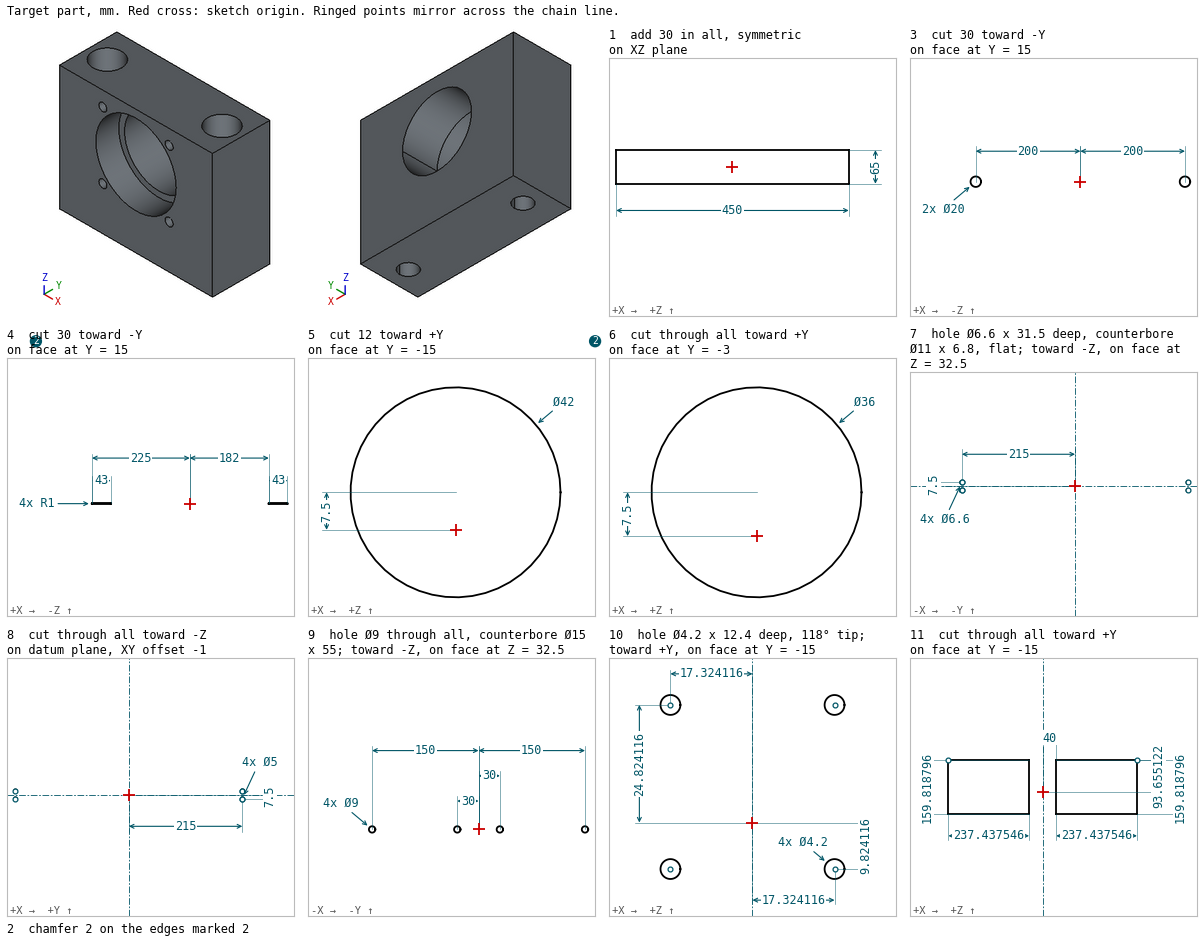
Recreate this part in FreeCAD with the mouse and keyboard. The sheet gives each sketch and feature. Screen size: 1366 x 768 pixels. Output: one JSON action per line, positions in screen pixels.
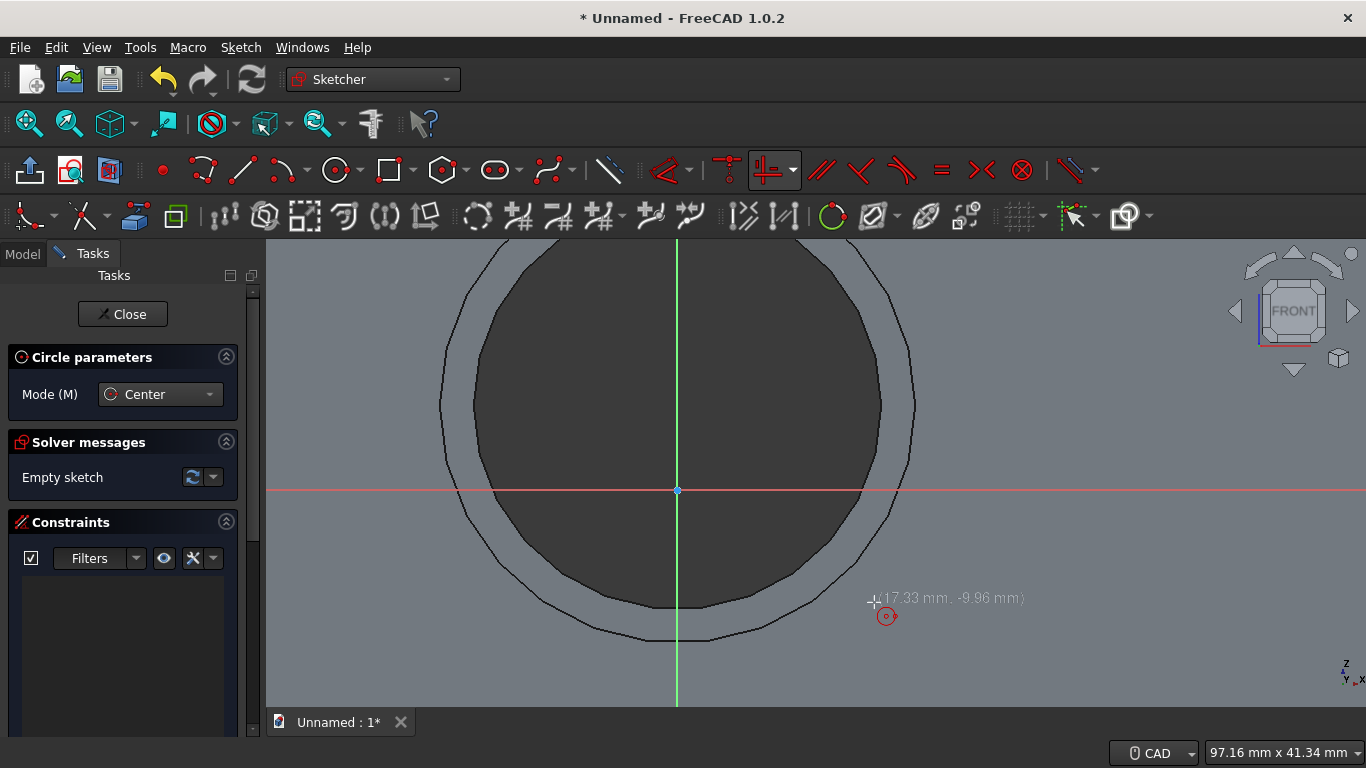
{"action": "left_click", "coordinate": [874, 602]}
{"action": "mouse_move", "coordinate": [890, 585]}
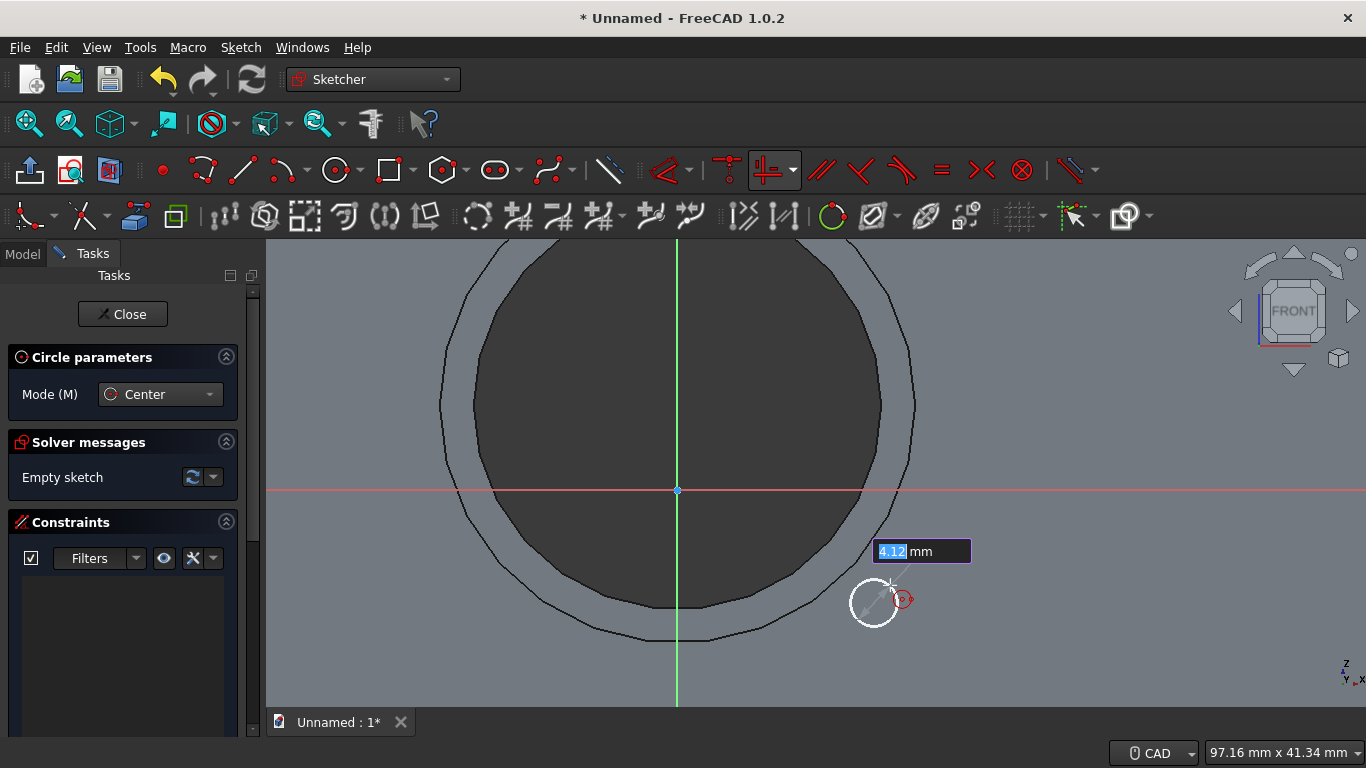
{"action": "type", "text": "4.2"}
{"action": "key", "text": "Return"}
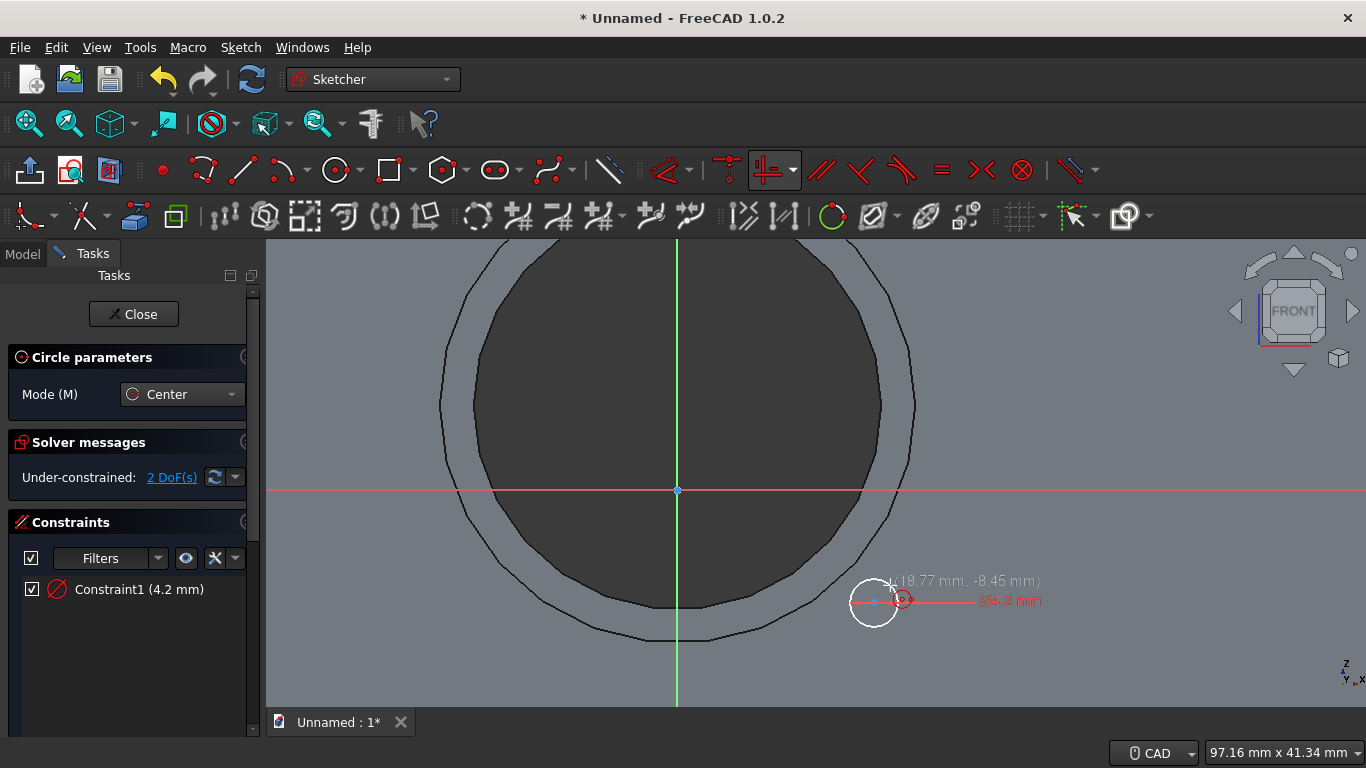
{"action": "left_click", "coordinate": [481, 602]}
{"action": "mouse_move", "coordinate": [498, 585]}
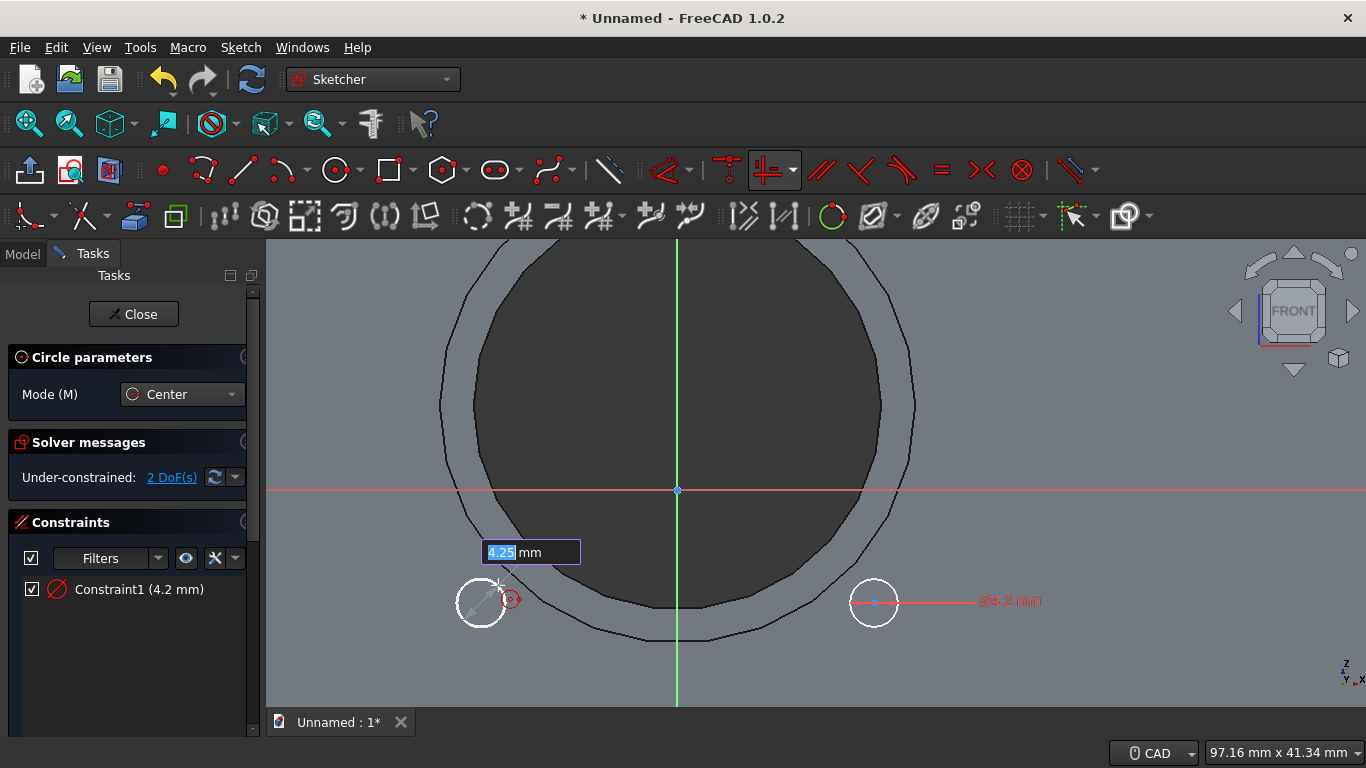
{"action": "type", "text": "4.2"}
{"action": "key", "text": "Return"}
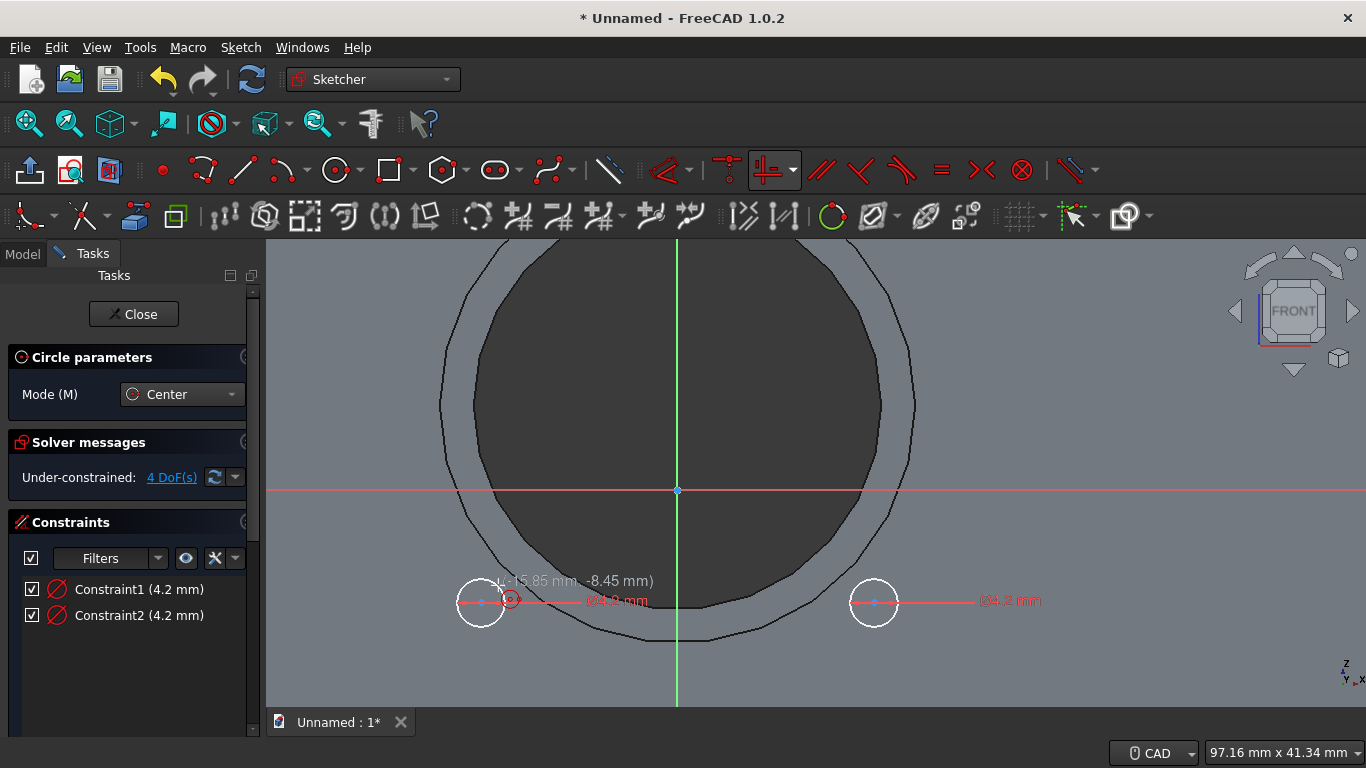
{"action": "scroll", "coordinate": [890, 610], "scroll_direction": "down", "scroll_amount": 2}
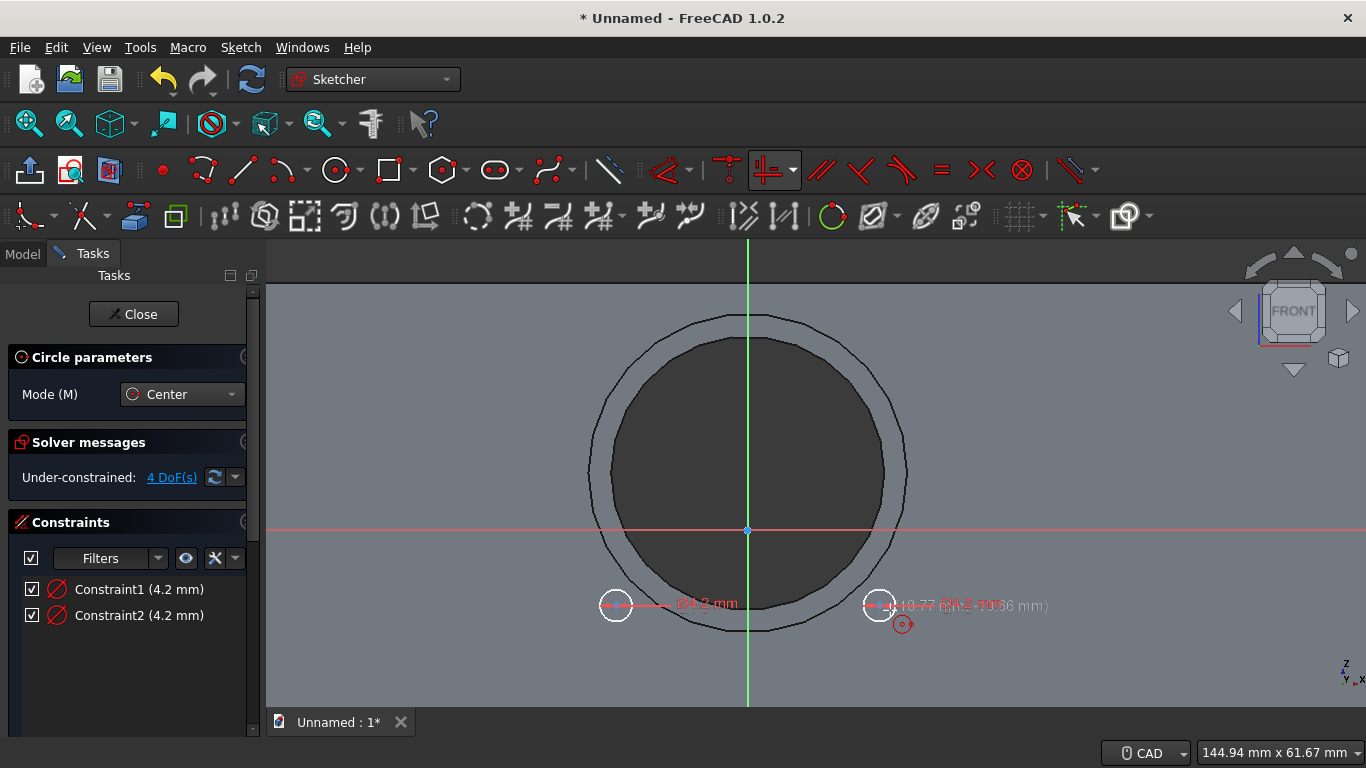
{"action": "scroll", "coordinate": [616, 342], "scroll_direction": "up", "scroll_amount": 2}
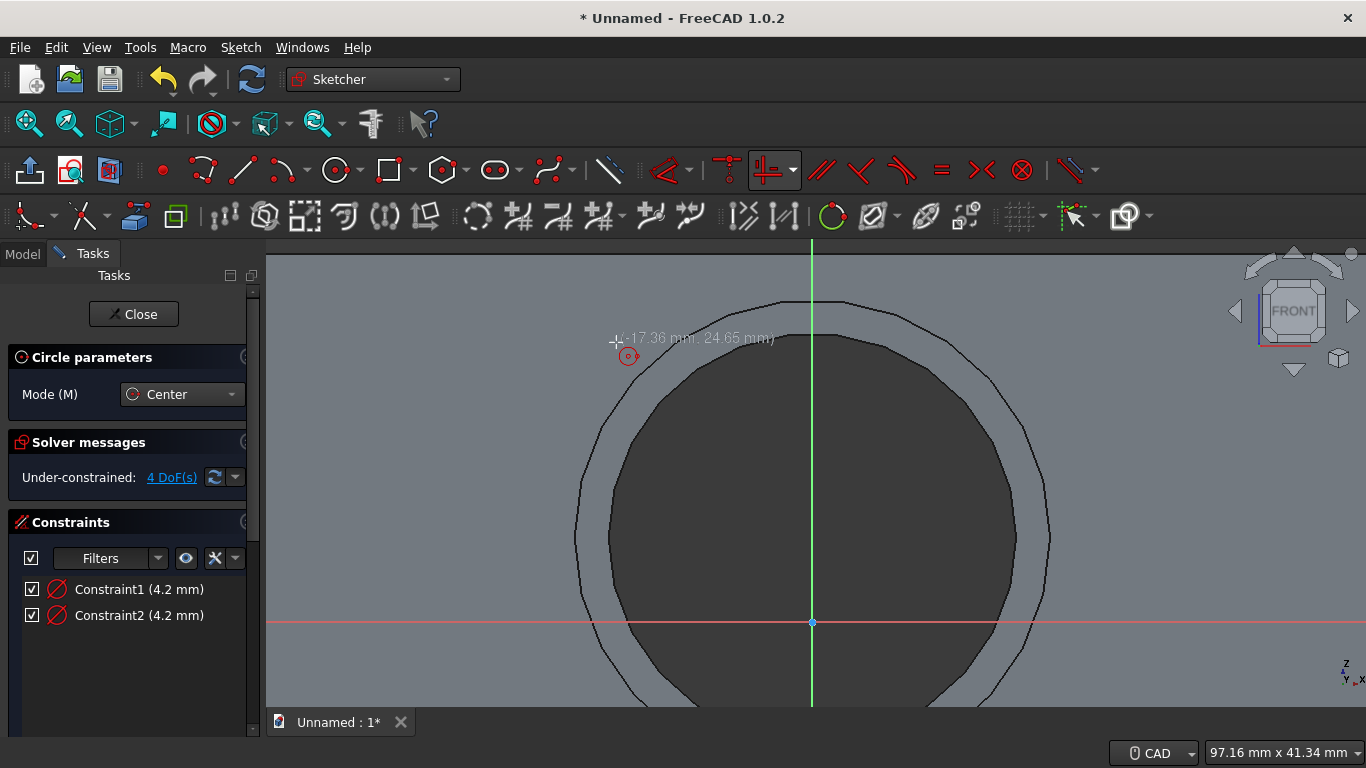
{"action": "left_click", "coordinate": [616, 341]}
{"action": "mouse_move", "coordinate": [633, 325]}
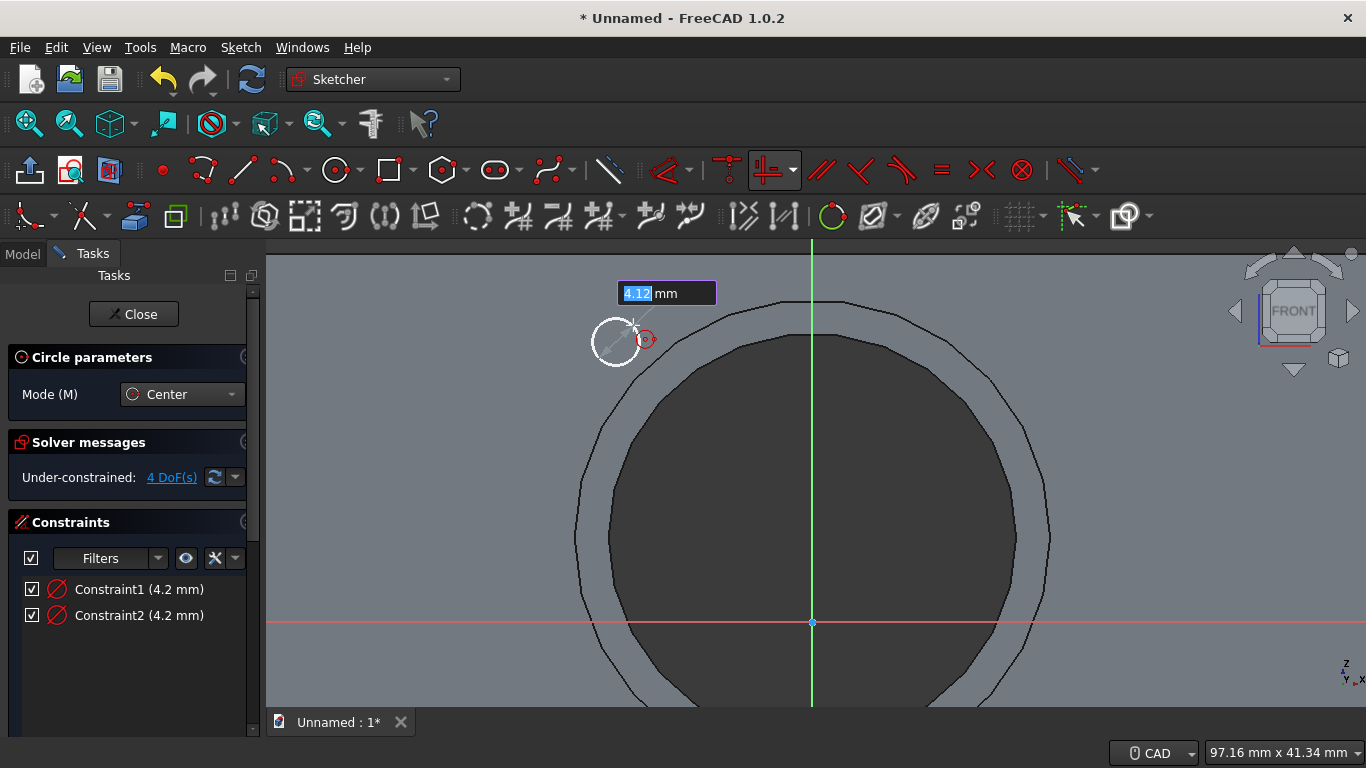
{"action": "type", "text": "4.2"}
{"action": "key", "text": "Return"}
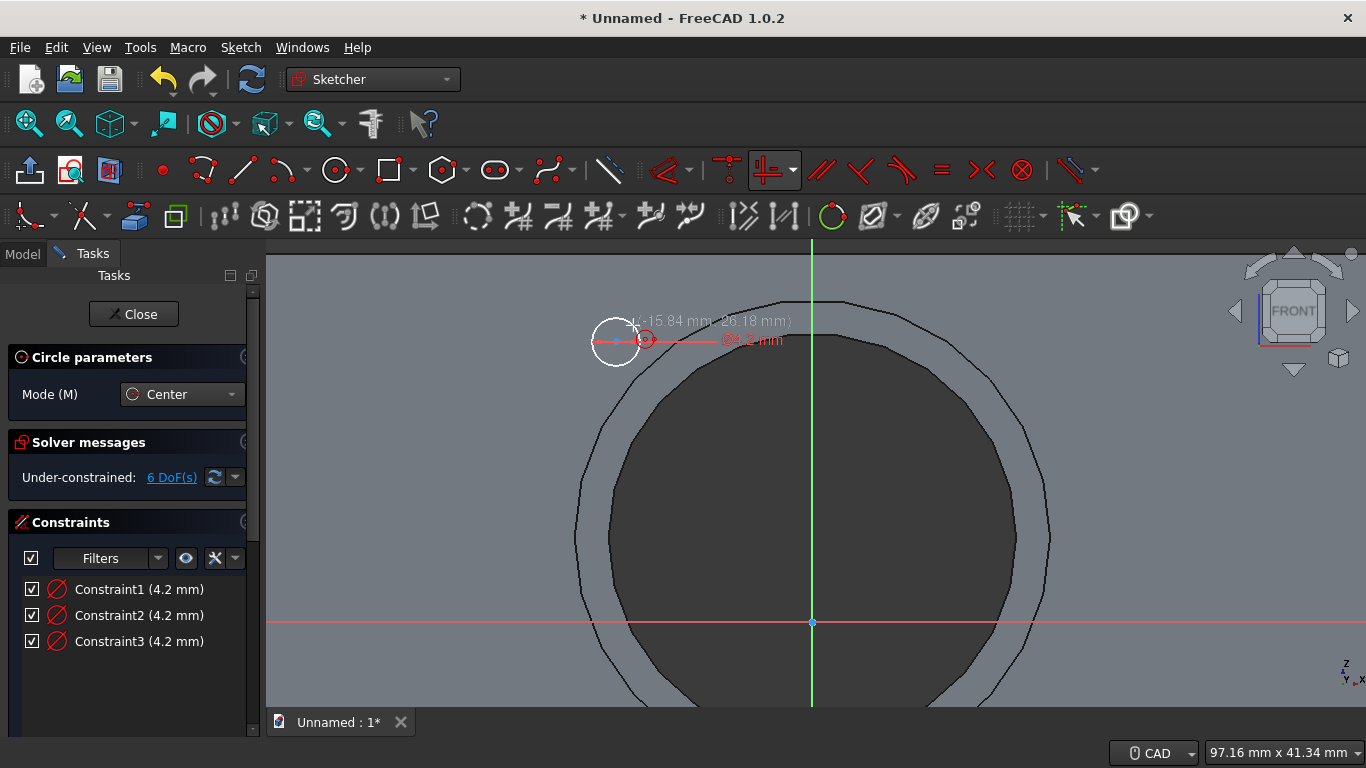
{"action": "left_click", "coordinate": [1009, 341]}
{"action": "mouse_move", "coordinate": [1025, 325]}